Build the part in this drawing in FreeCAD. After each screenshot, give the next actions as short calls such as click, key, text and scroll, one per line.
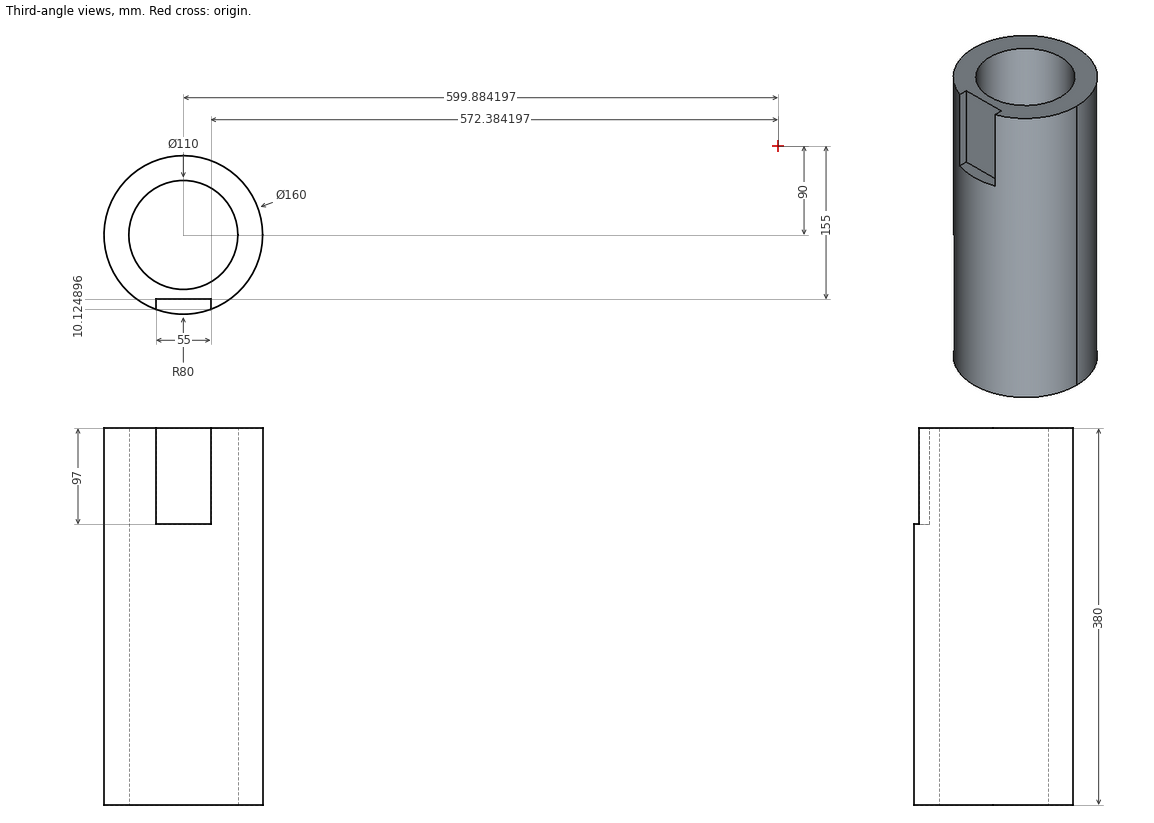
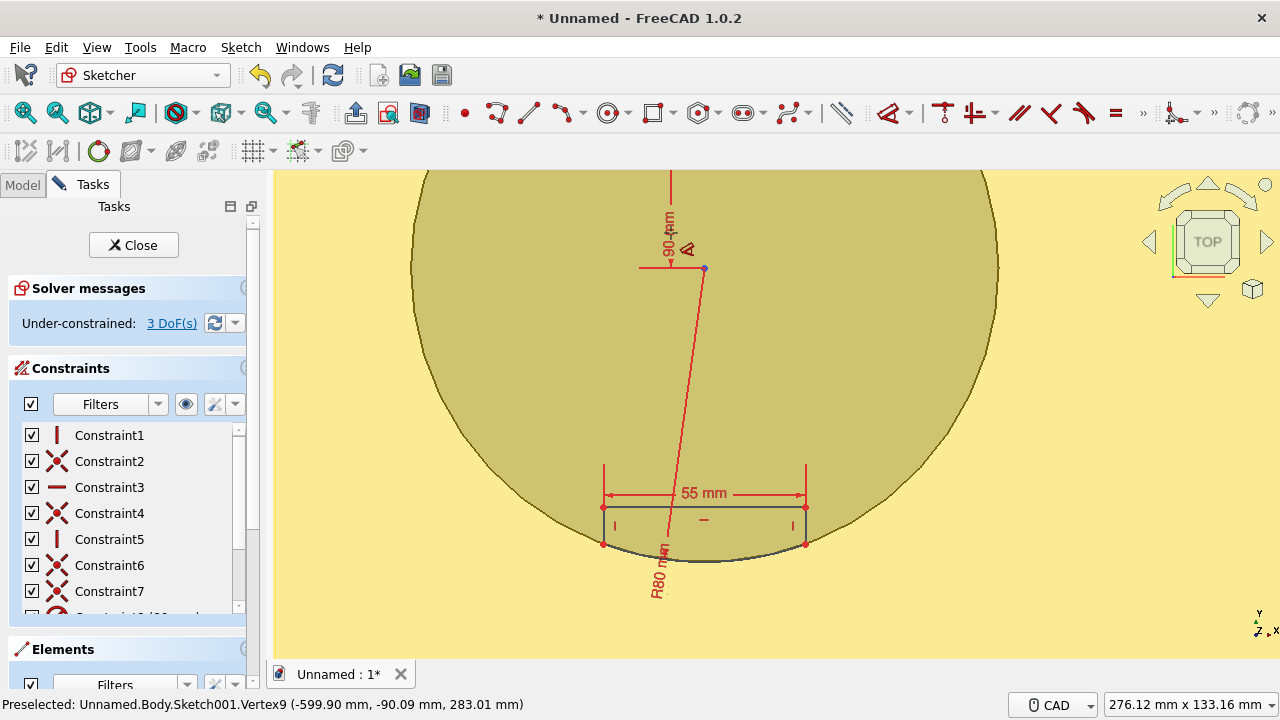
click(806, 507)
click(772, 353)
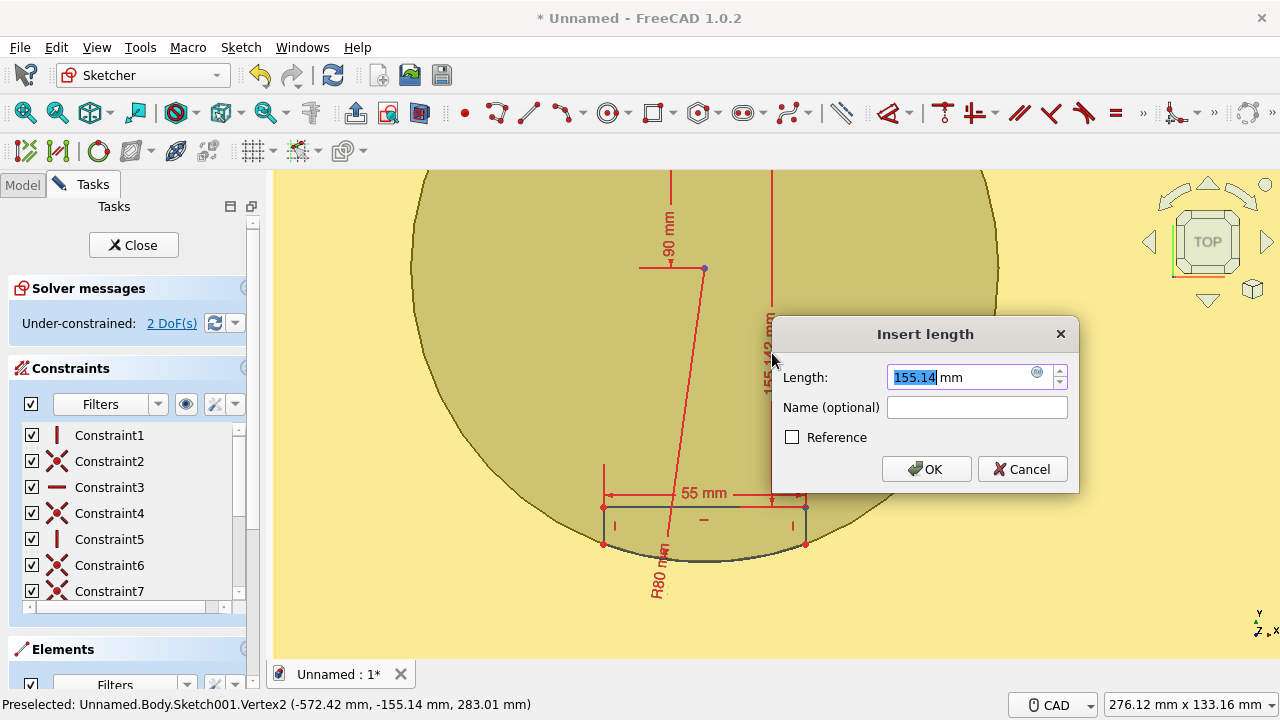
text(155)
key(Return)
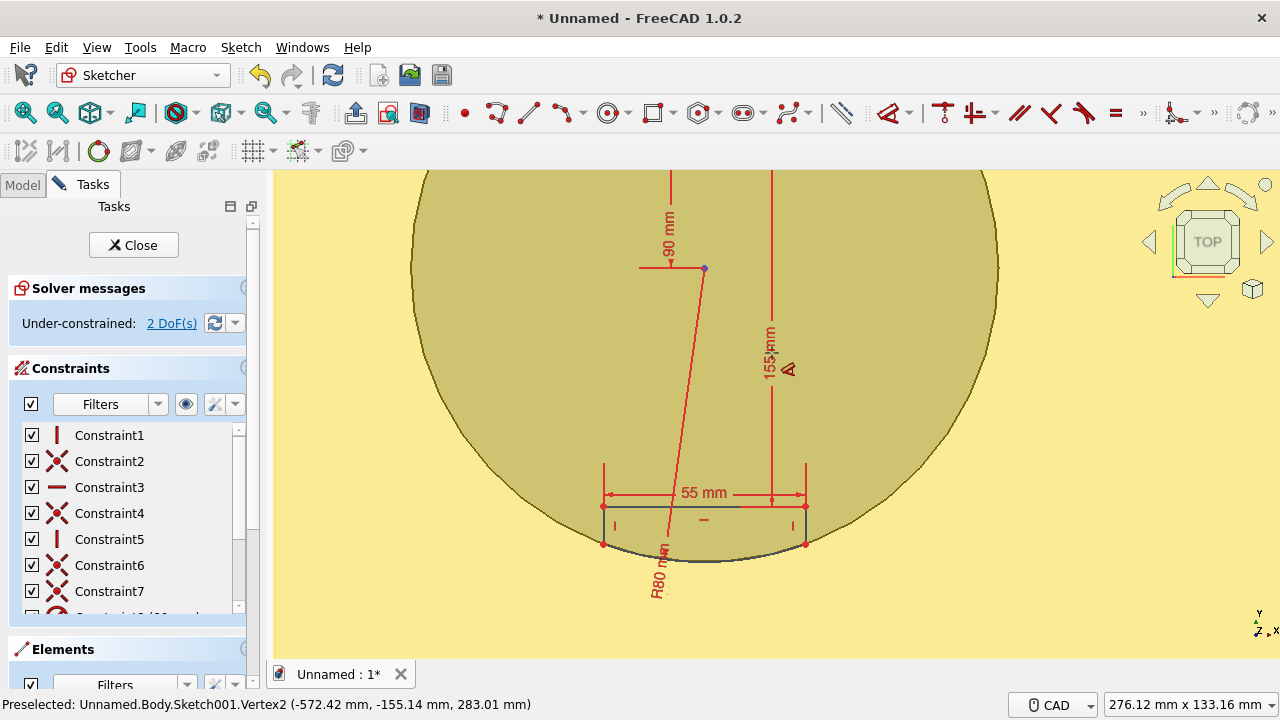
scroll(806, 533, up, 2)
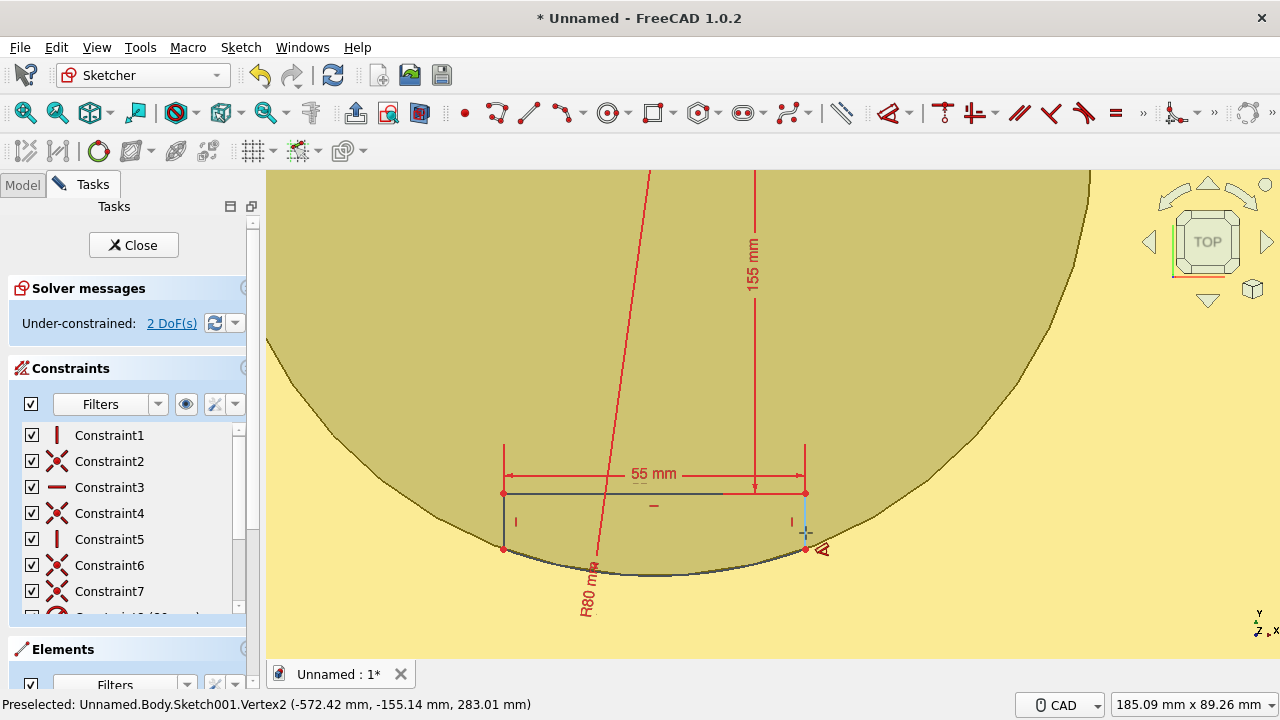
click(805, 533)
click(839, 521)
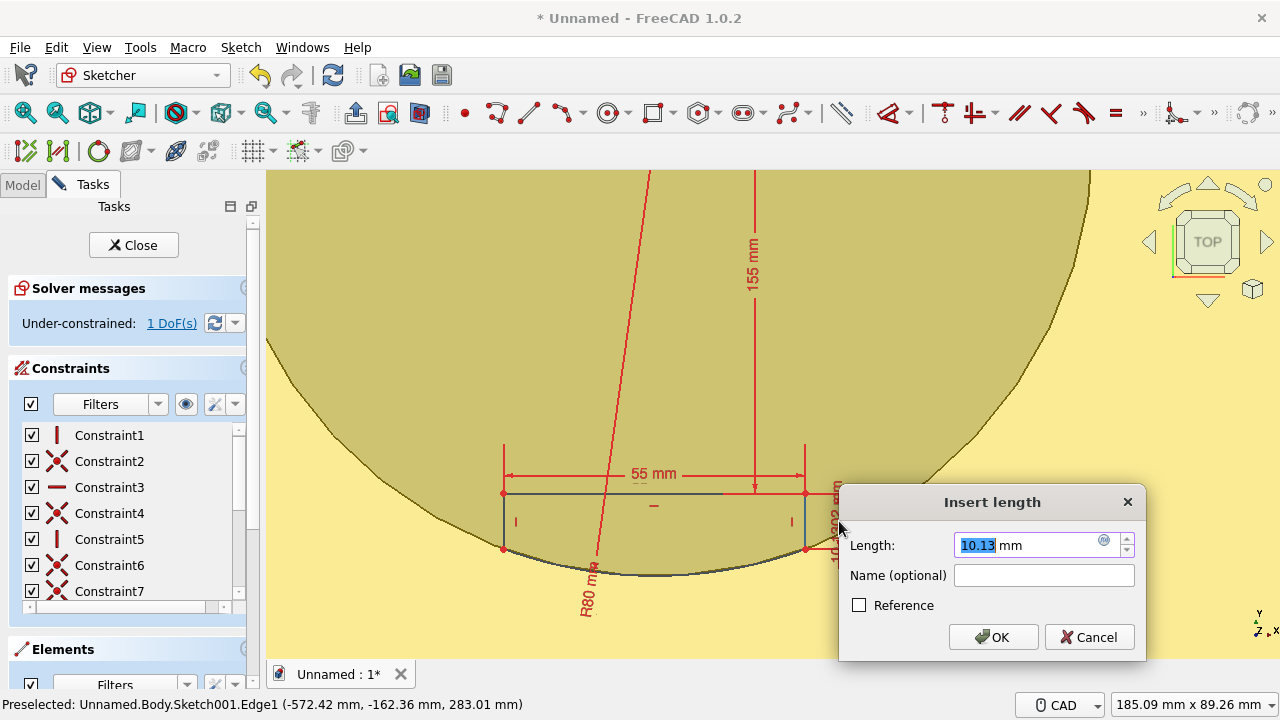
text(10.124896)
key(Return)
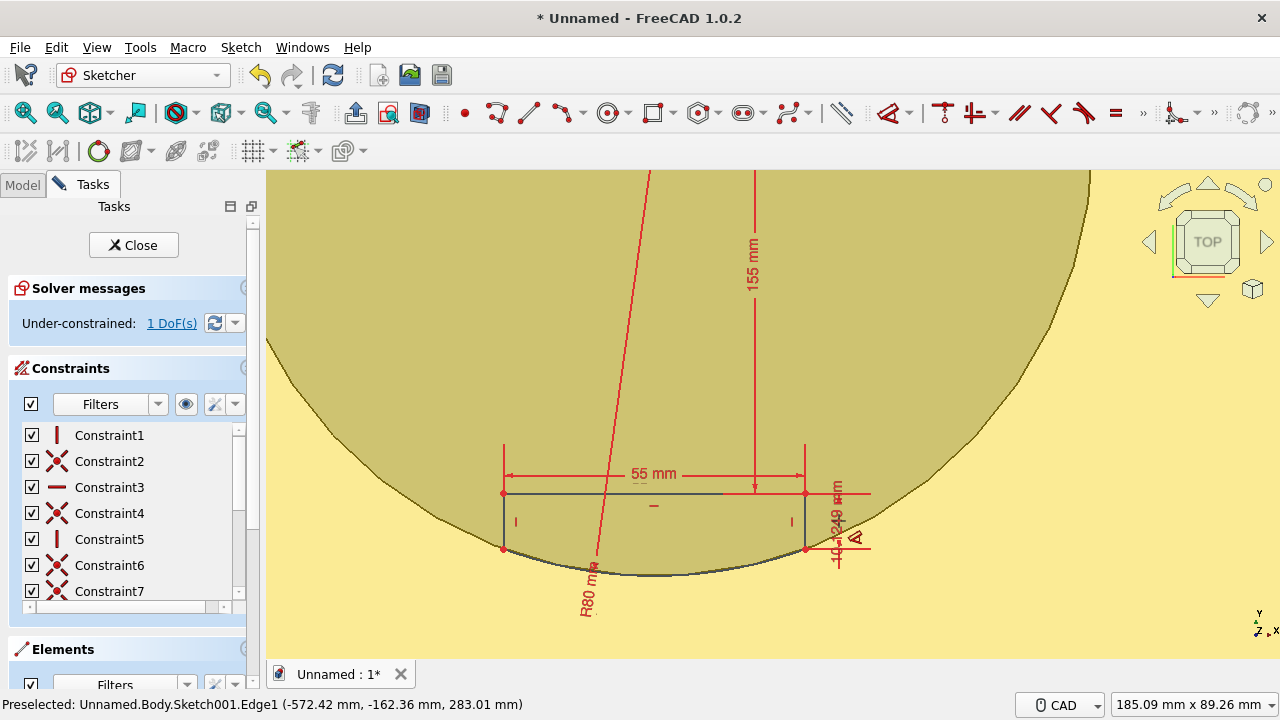
click(805, 549)
click(960, 583)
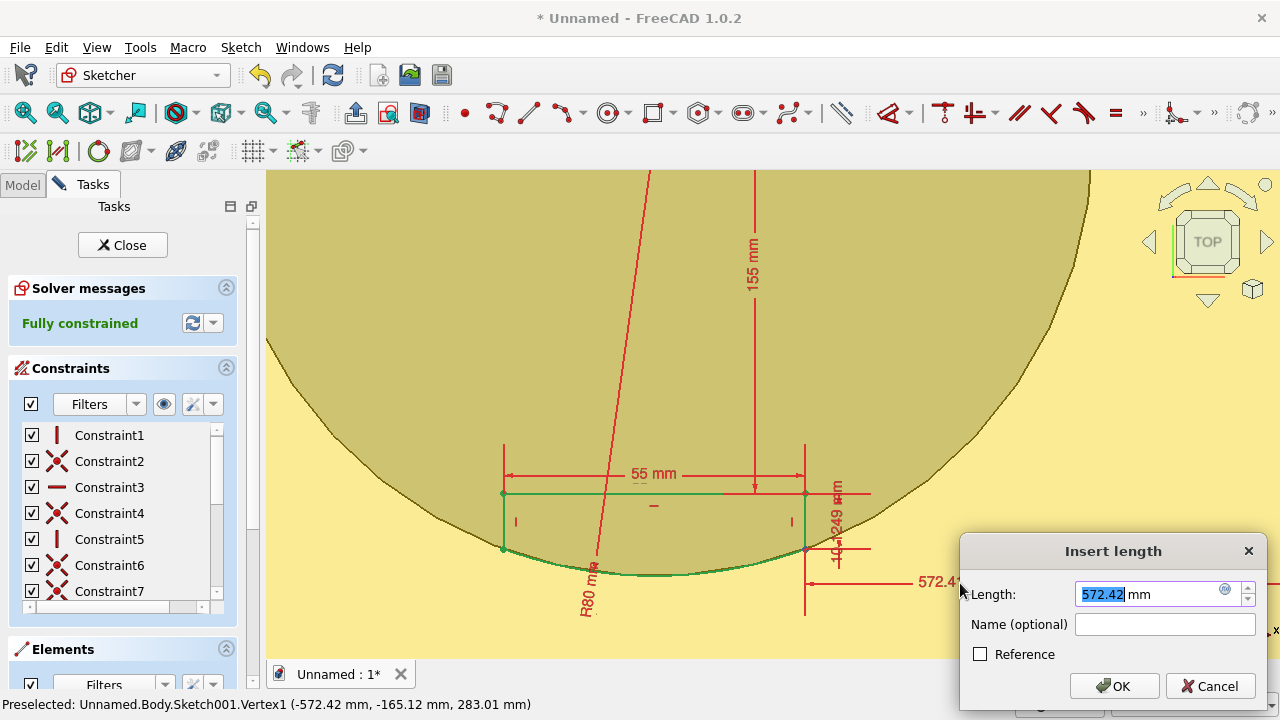
text(572.384197)
key(Return)
key(Escape)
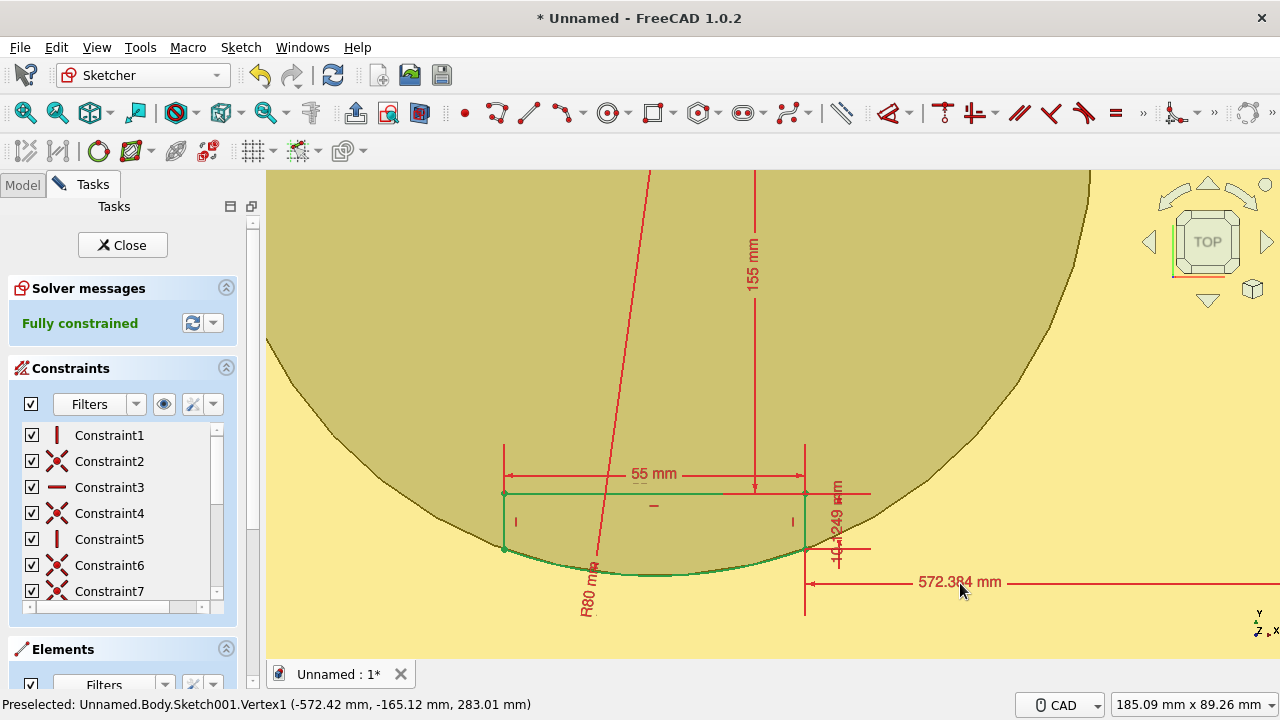
click(123, 245)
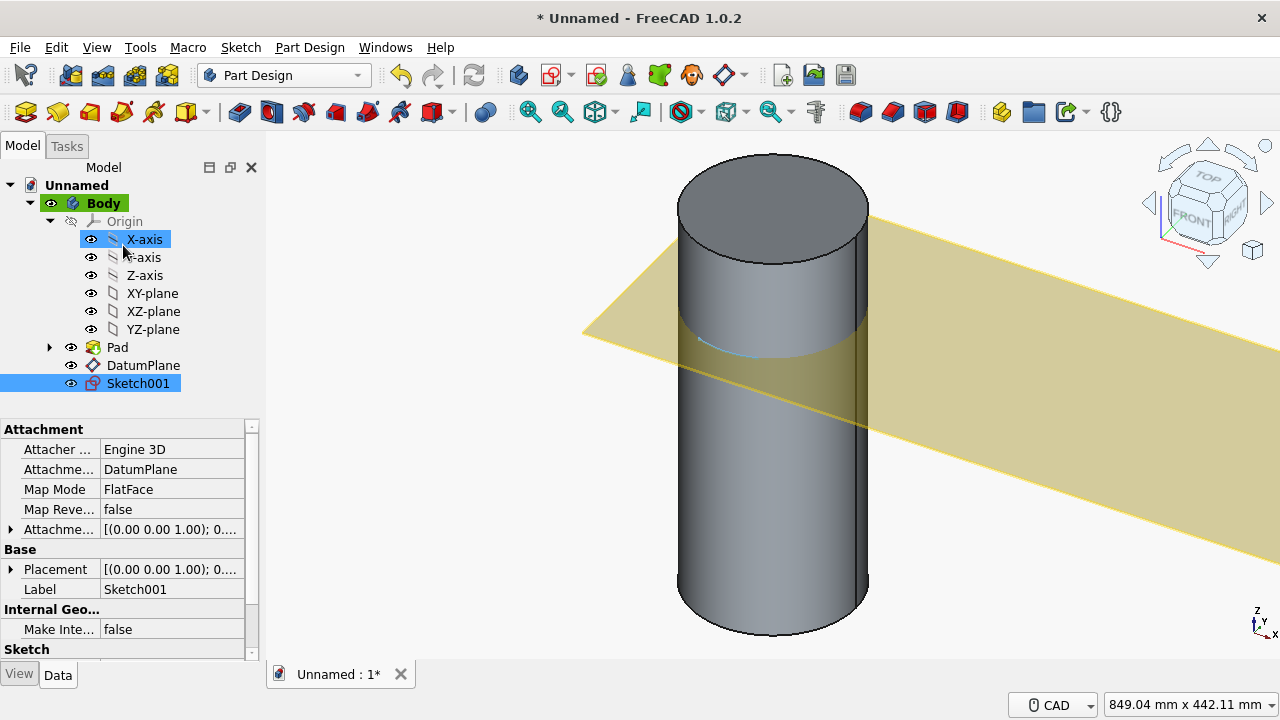
click(240, 112)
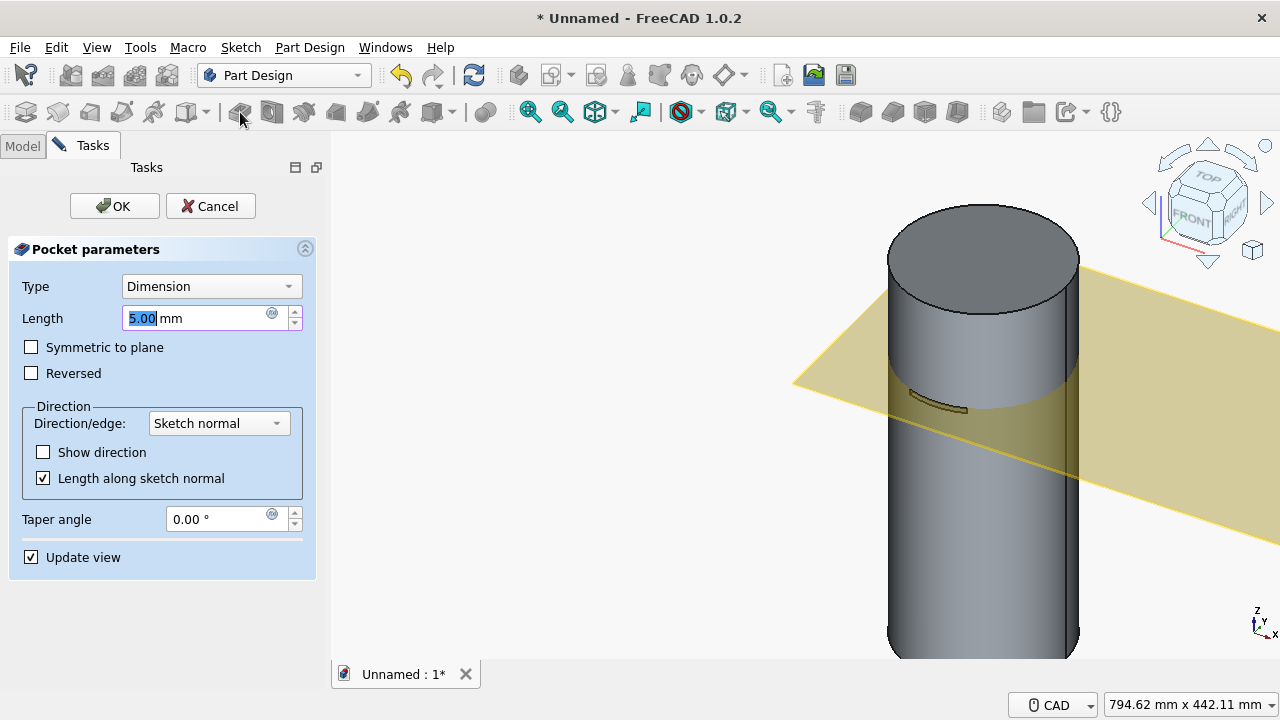
text(97)
key(Tab)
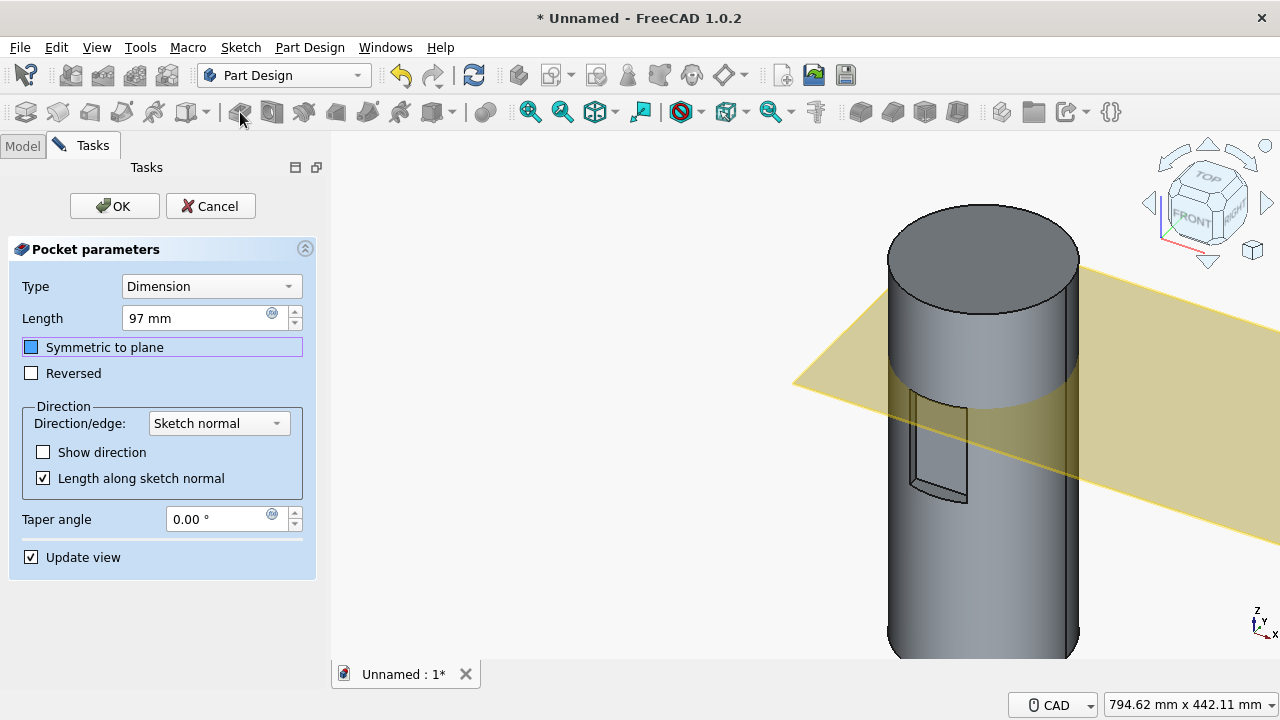
click(30, 373)